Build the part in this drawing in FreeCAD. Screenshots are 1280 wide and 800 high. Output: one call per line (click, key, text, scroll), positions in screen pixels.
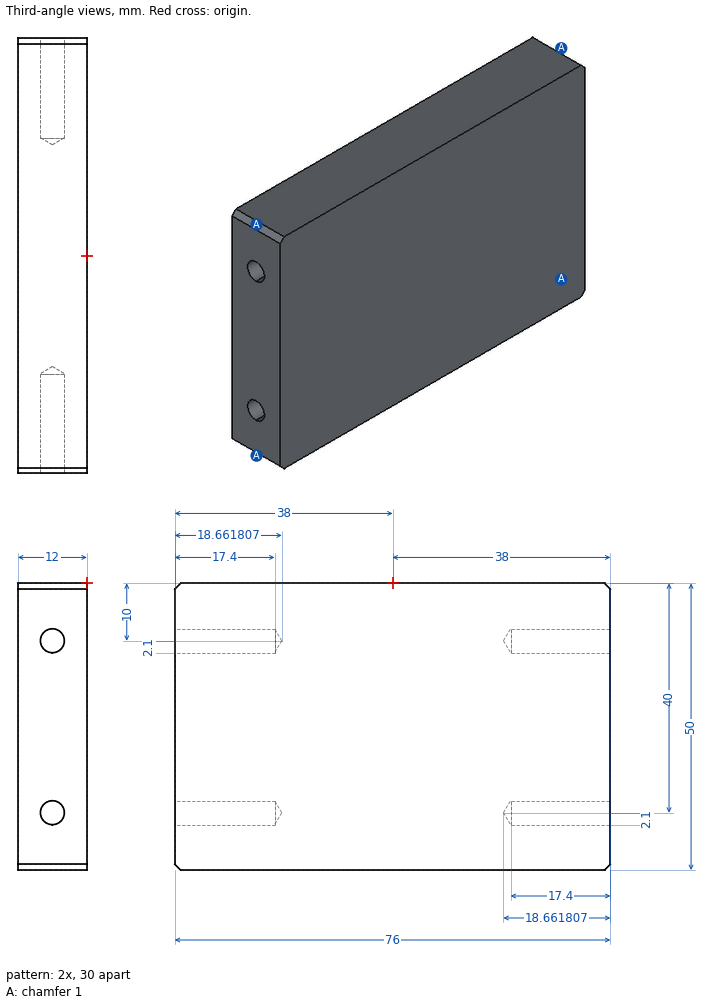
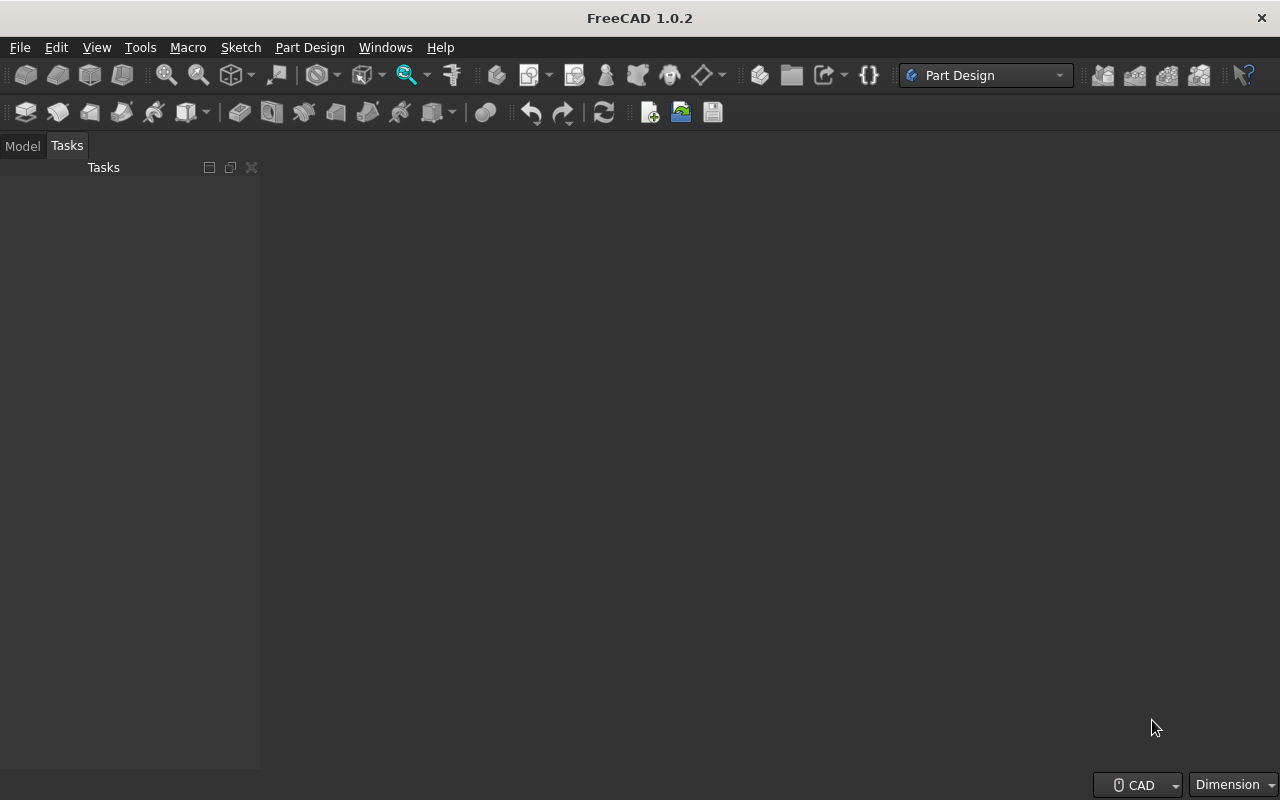
click(650, 112)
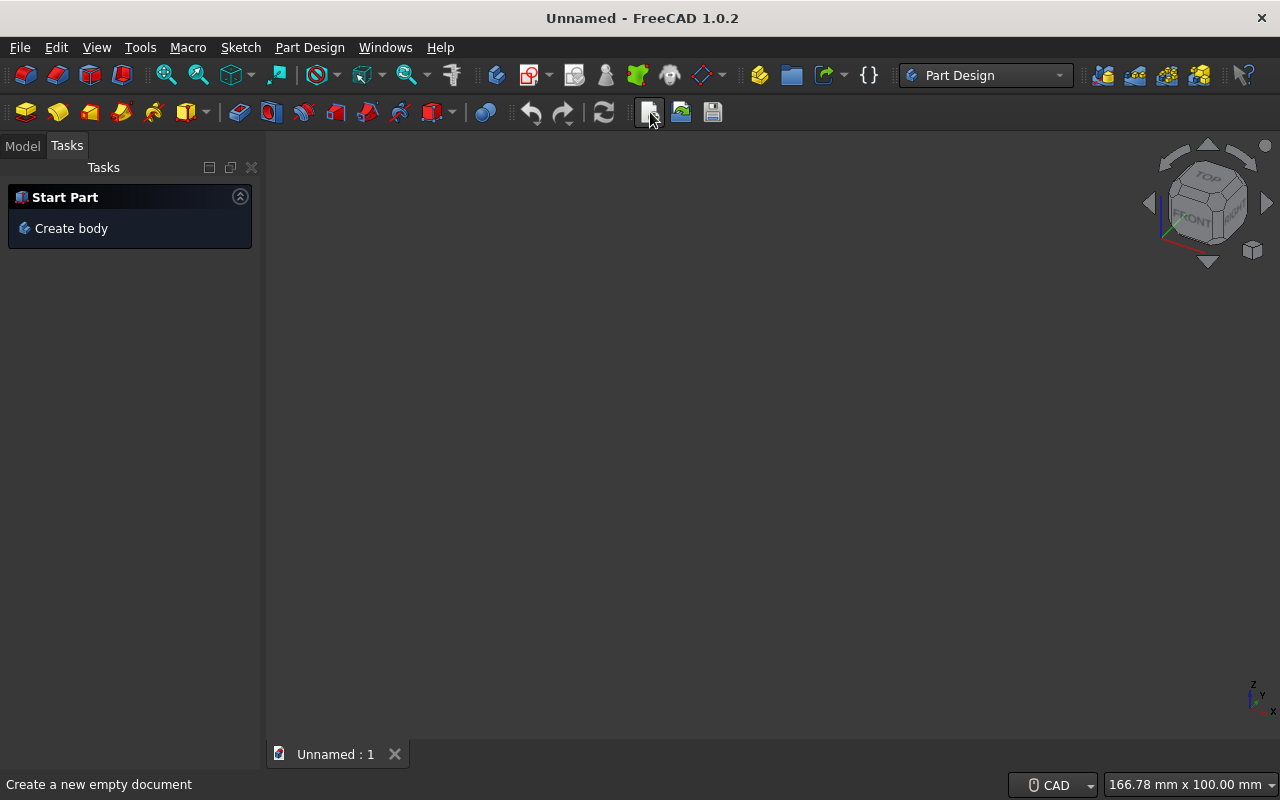
click(530, 76)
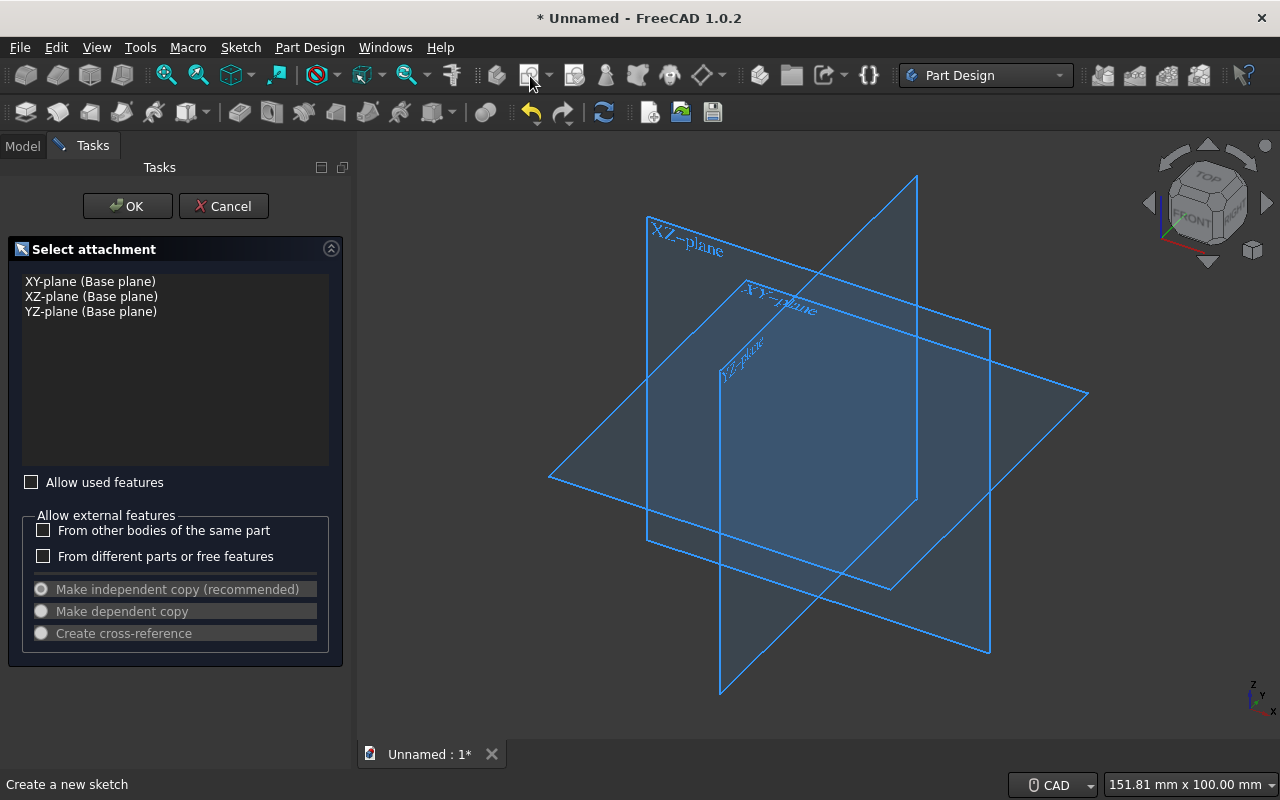
click(82, 312)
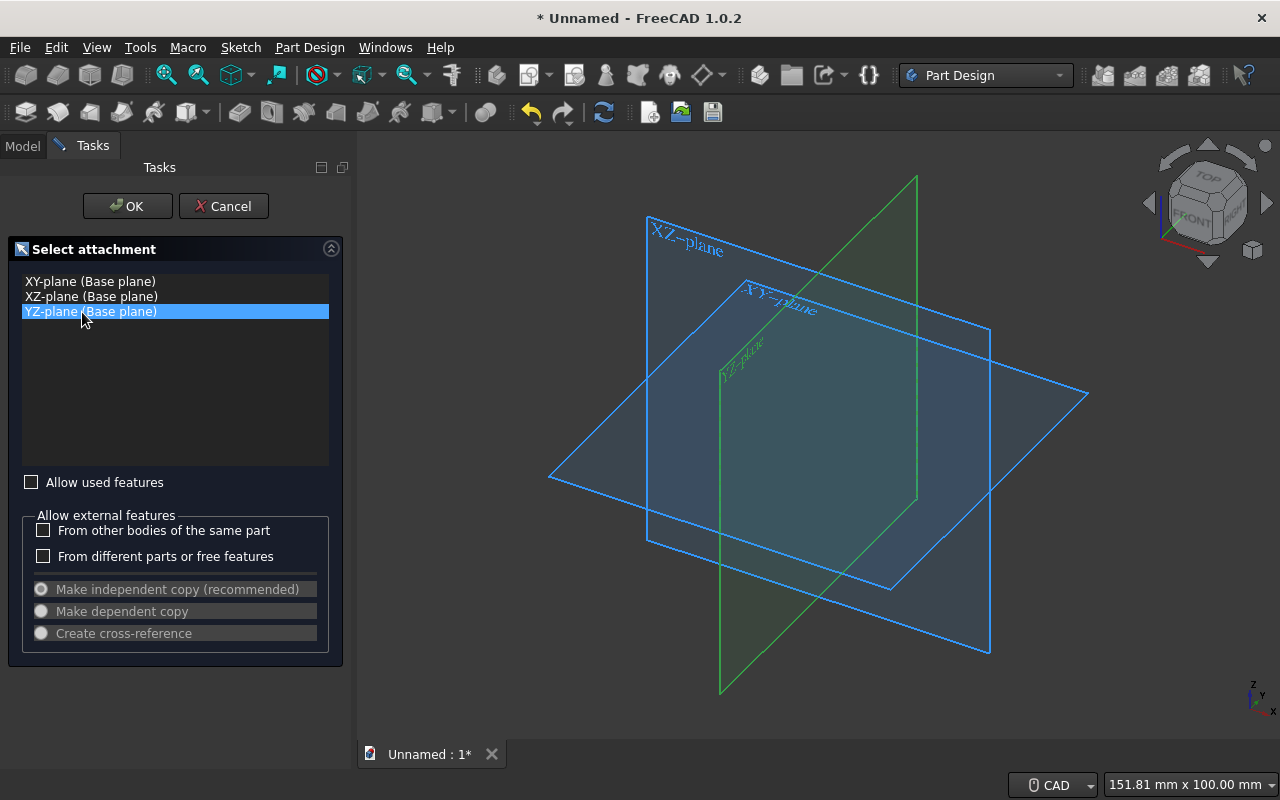
click(128, 206)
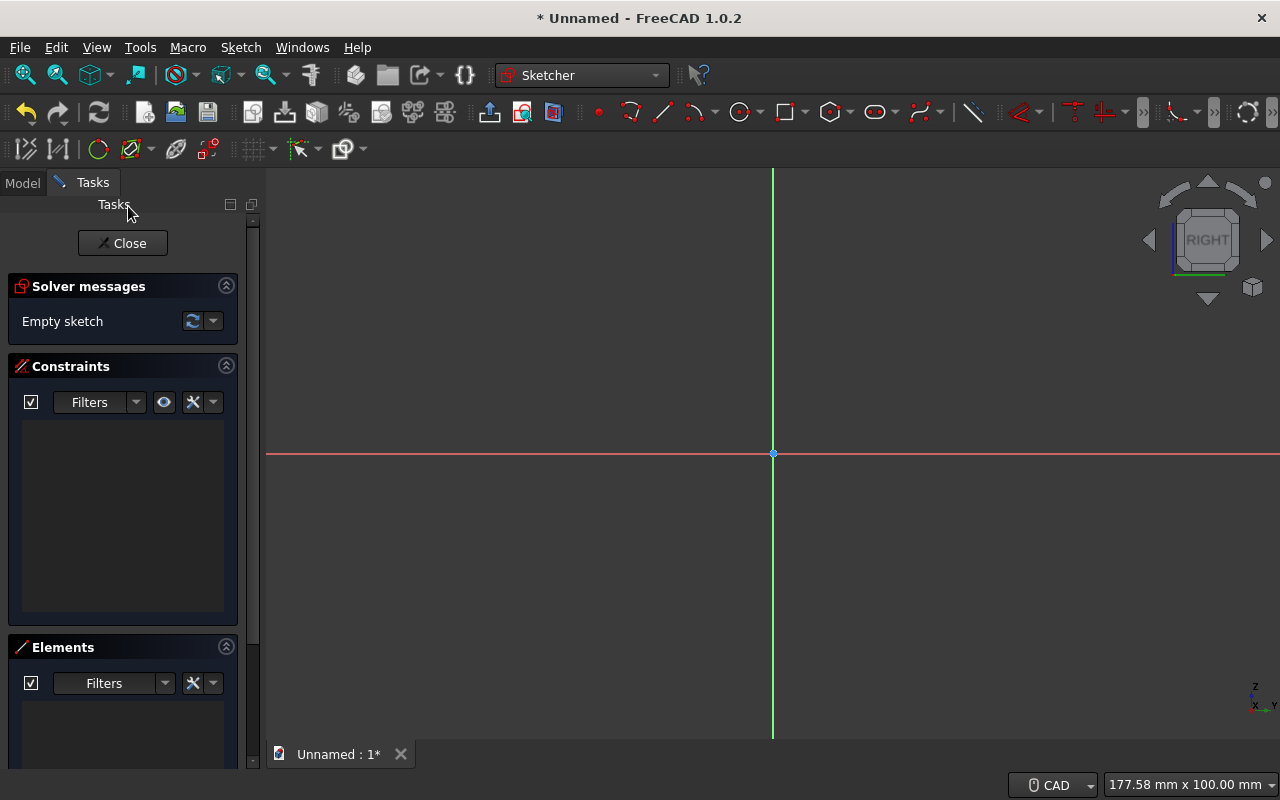
scroll(395, 196, down, 1)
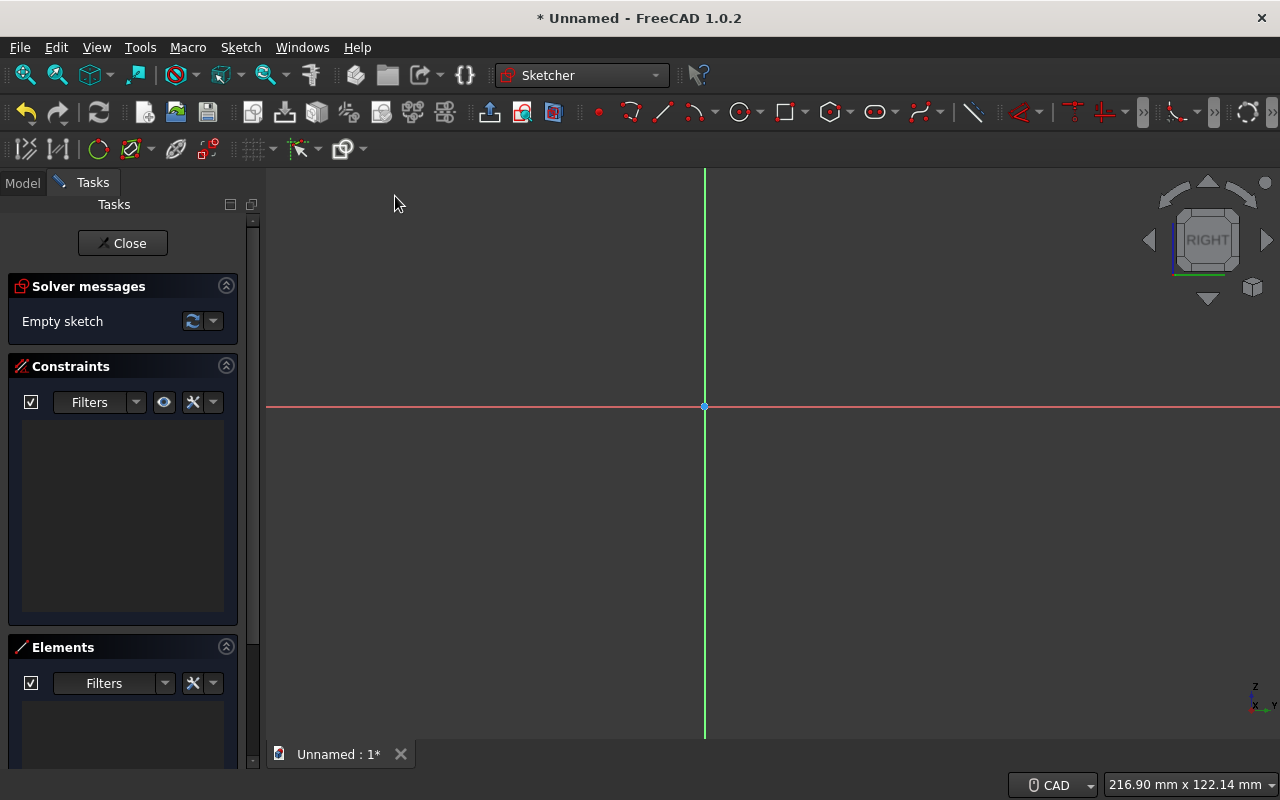
scroll(705, 666, up, 2)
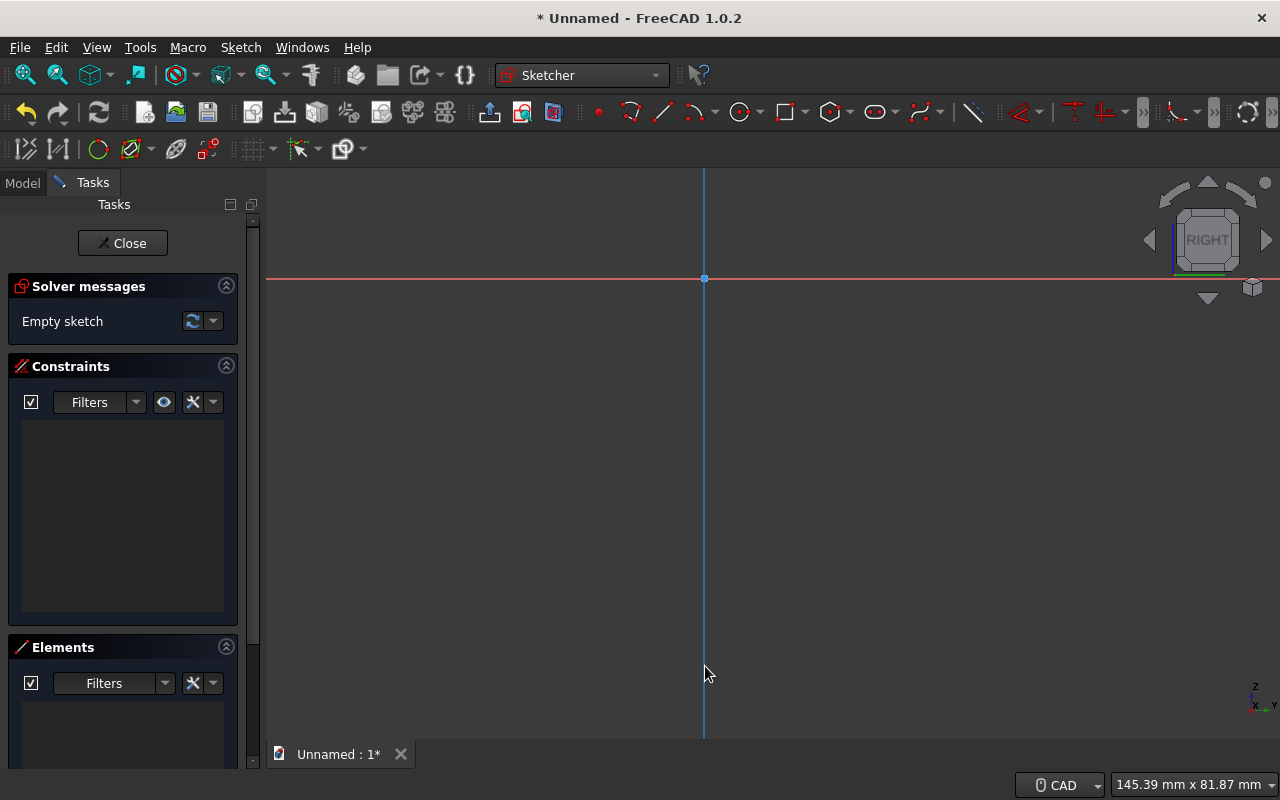
click(786, 112)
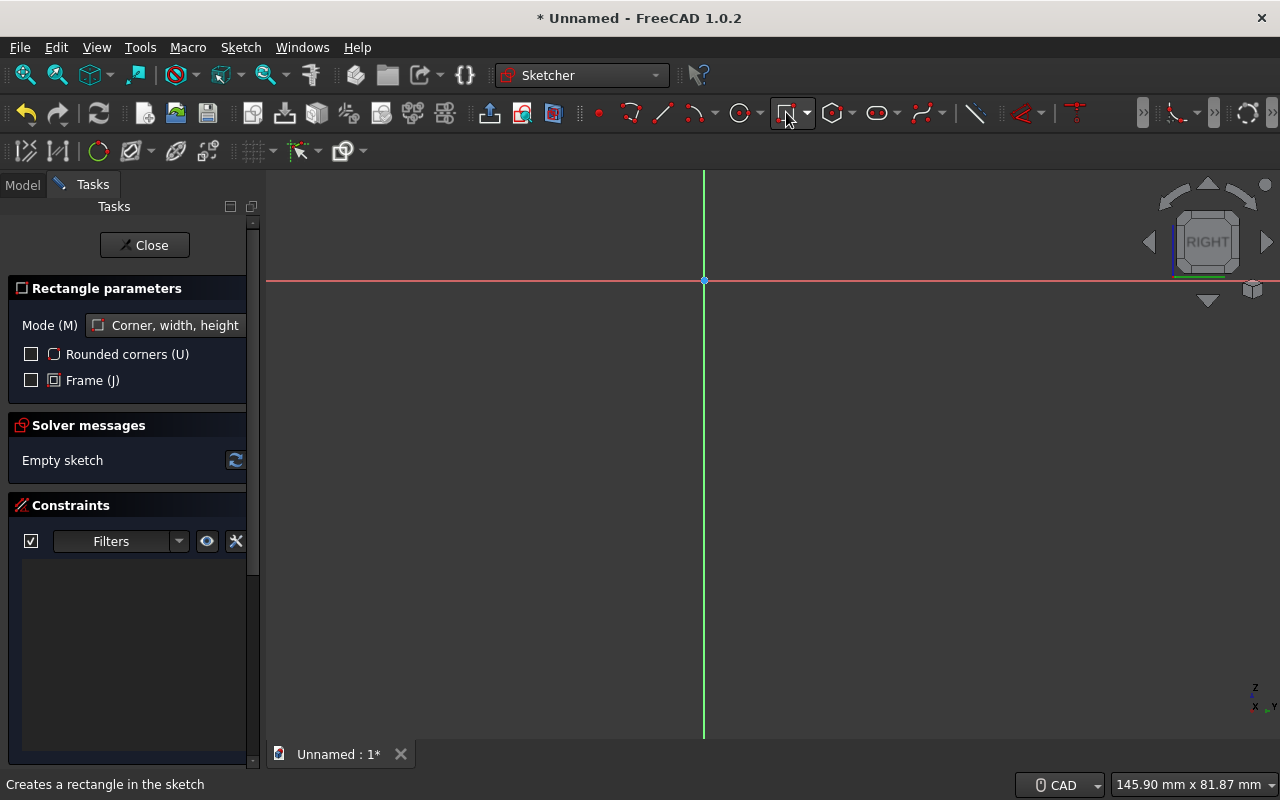
click(440, 281)
move(968, 628)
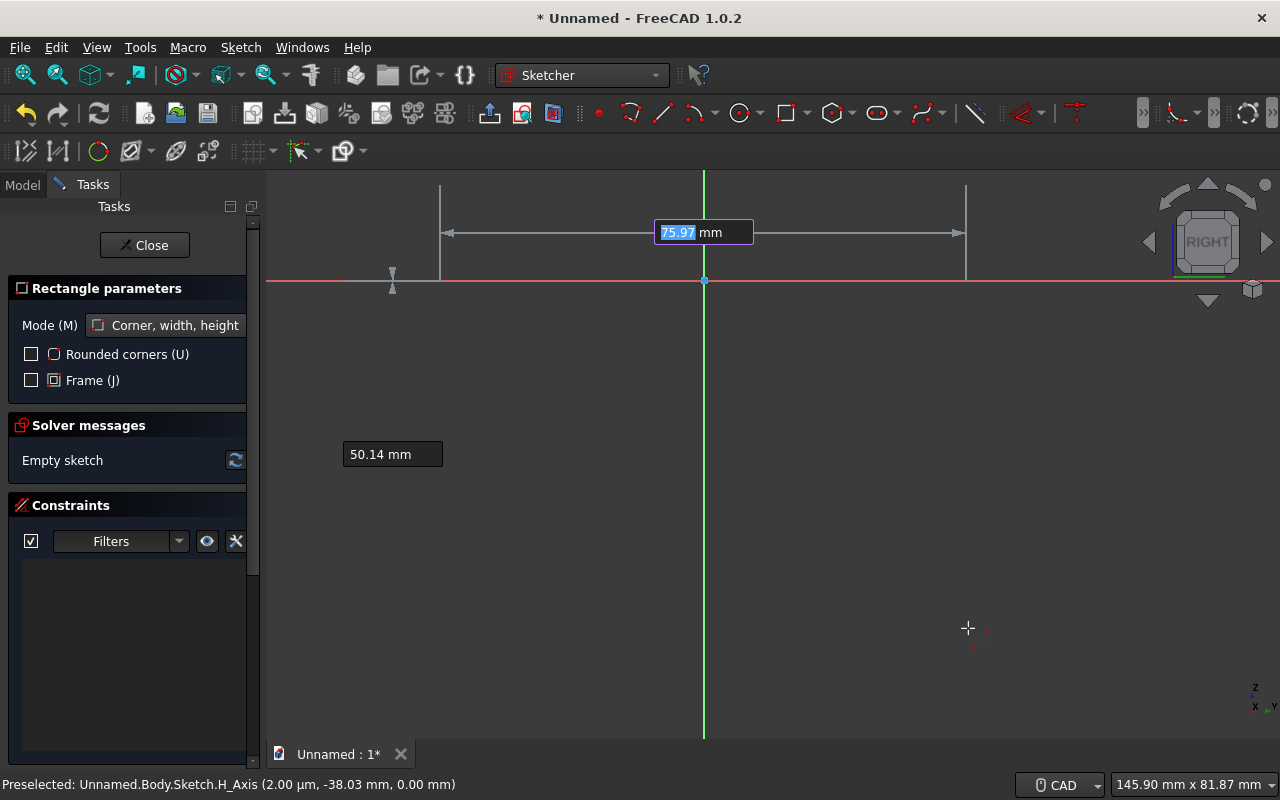
text(76)
key(Tab)
text(50)
key(Return)
key(Escape)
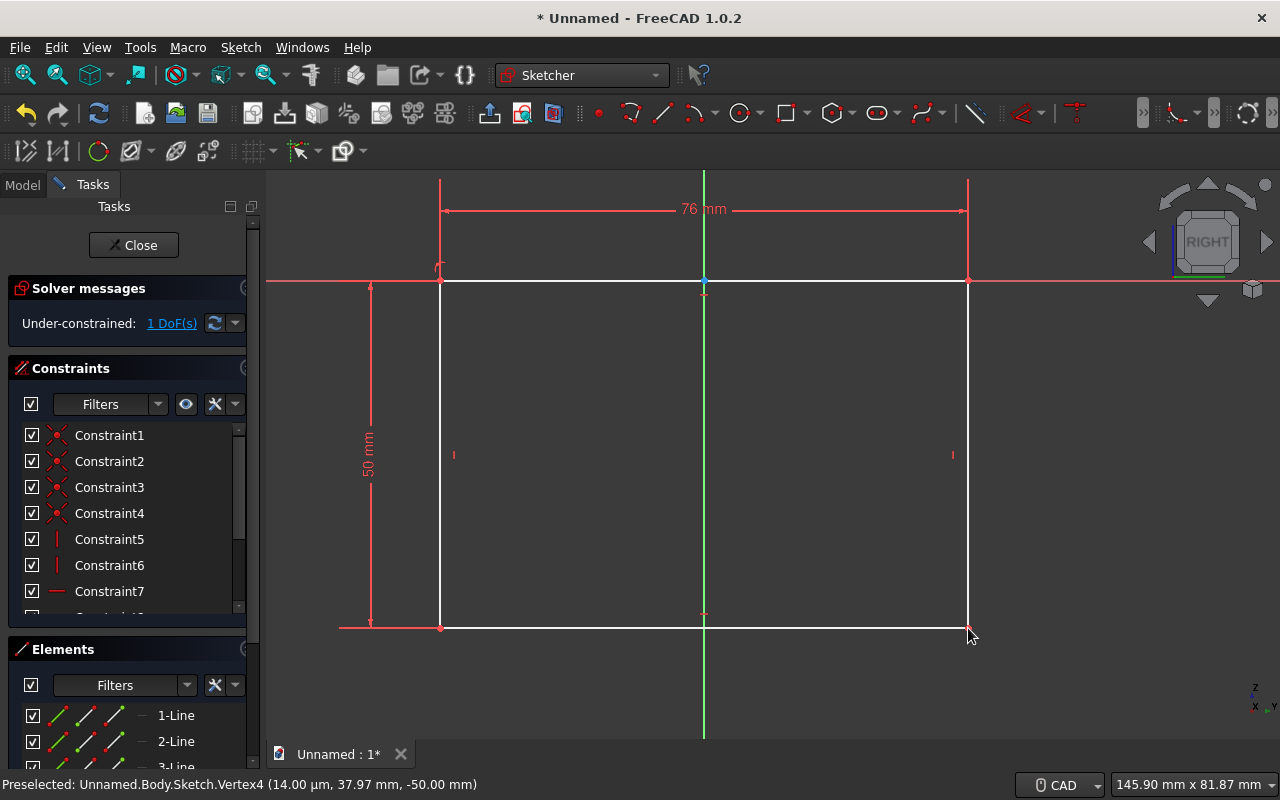
click(440, 281)